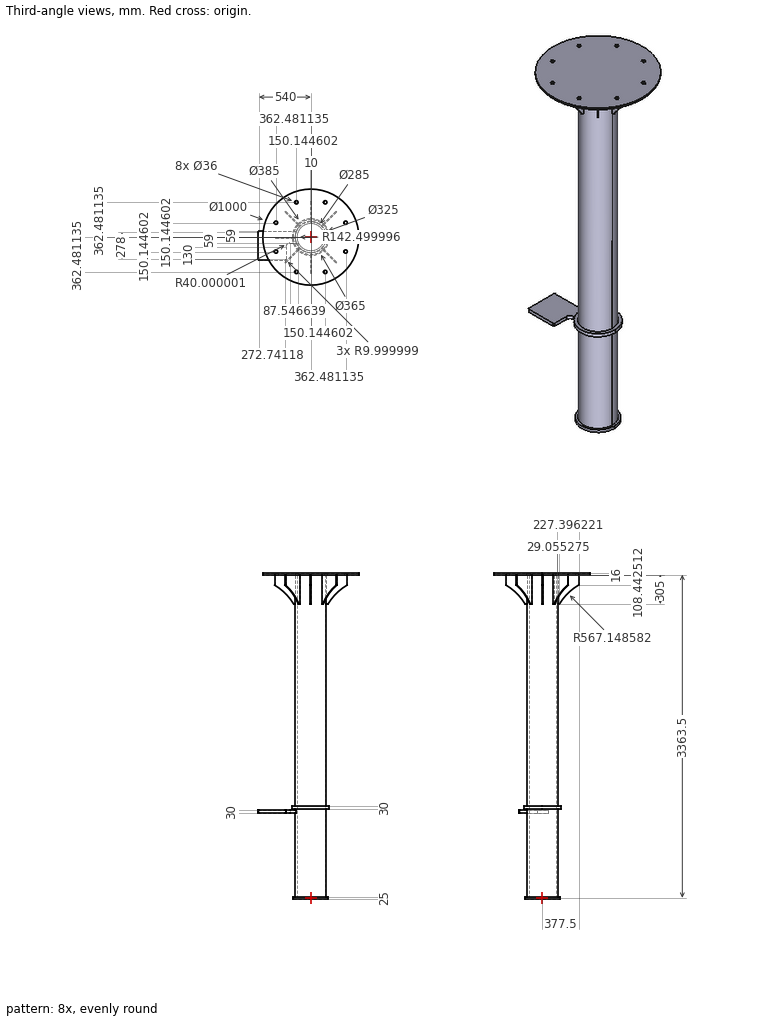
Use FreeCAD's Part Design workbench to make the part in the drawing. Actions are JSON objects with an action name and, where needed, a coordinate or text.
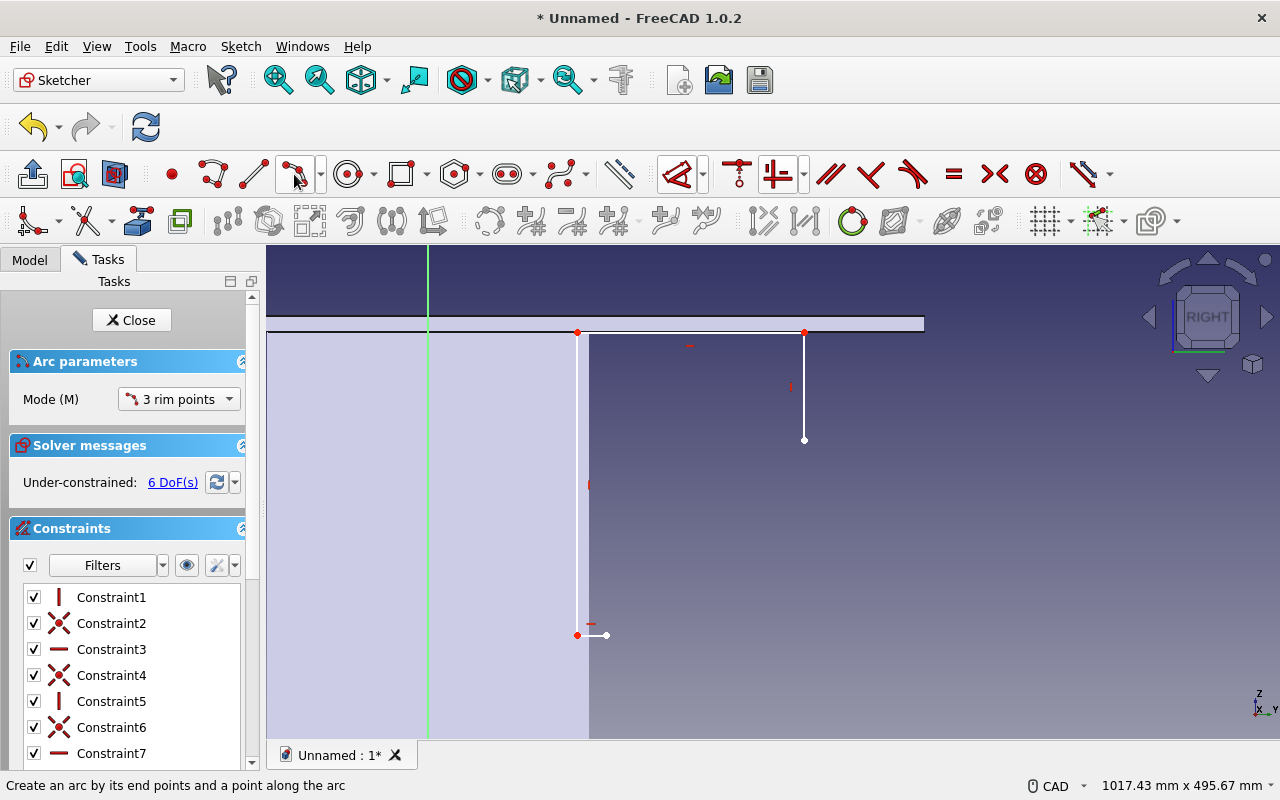
{"action": "left_click", "coordinate": [606, 636]}
{"action": "left_click", "coordinate": [804, 441]}
{"action": "left_click", "coordinate": [693, 525]}
{"action": "key", "text": "Escape"}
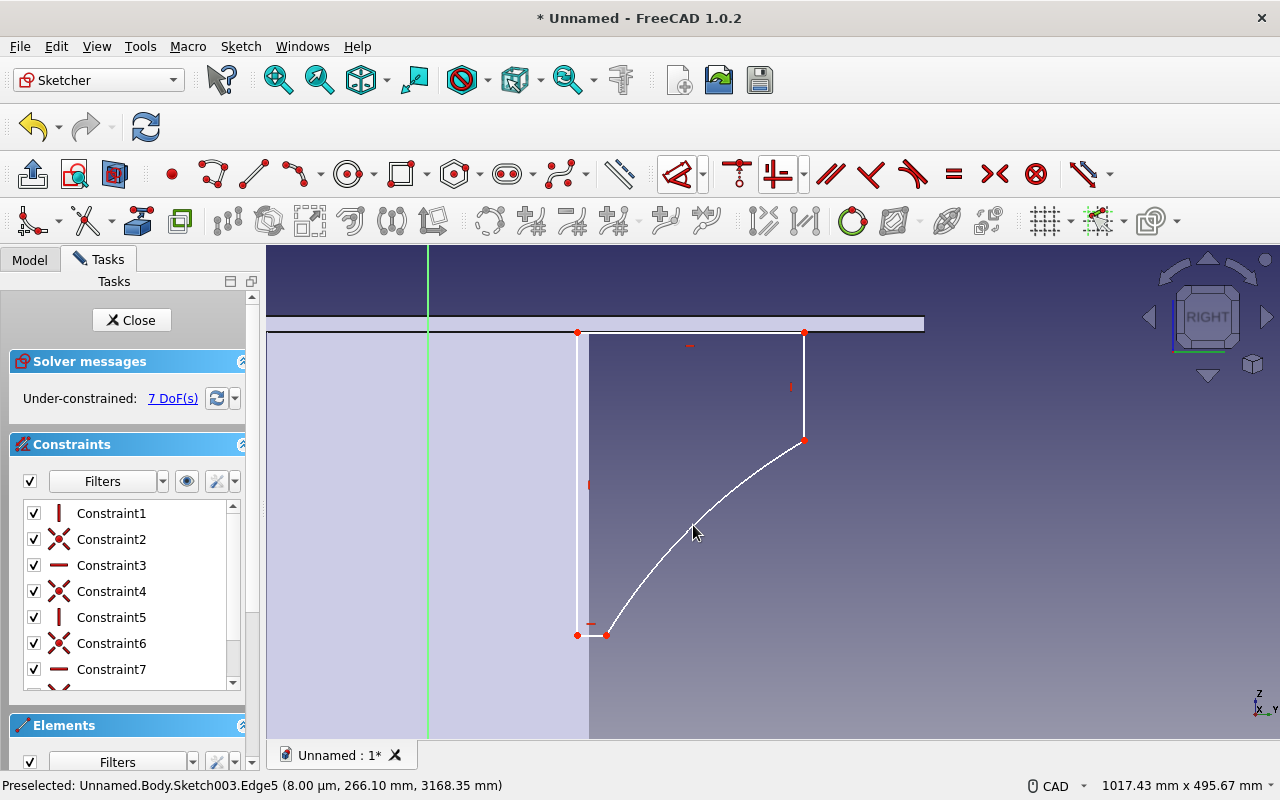
{"action": "left_click", "coordinate": [735, 489]}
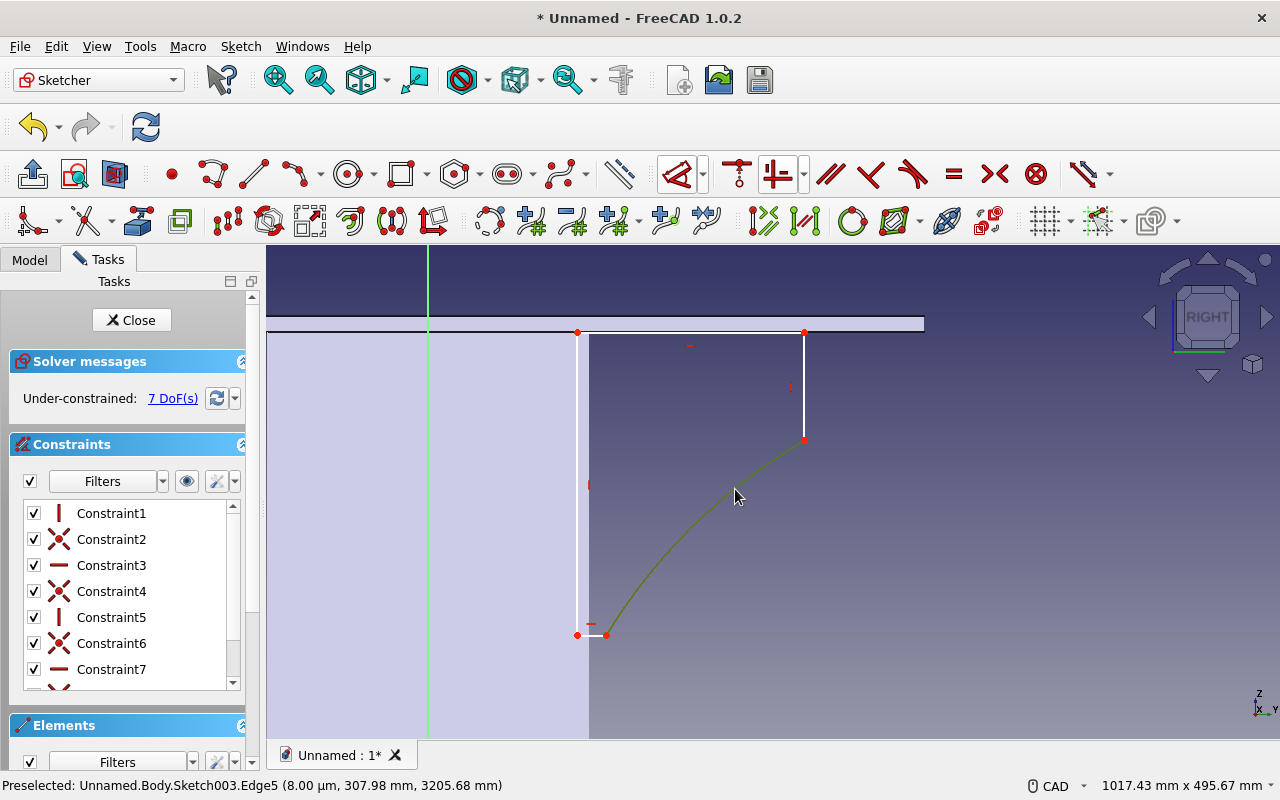
{"action": "left_click", "coordinate": [702, 174]}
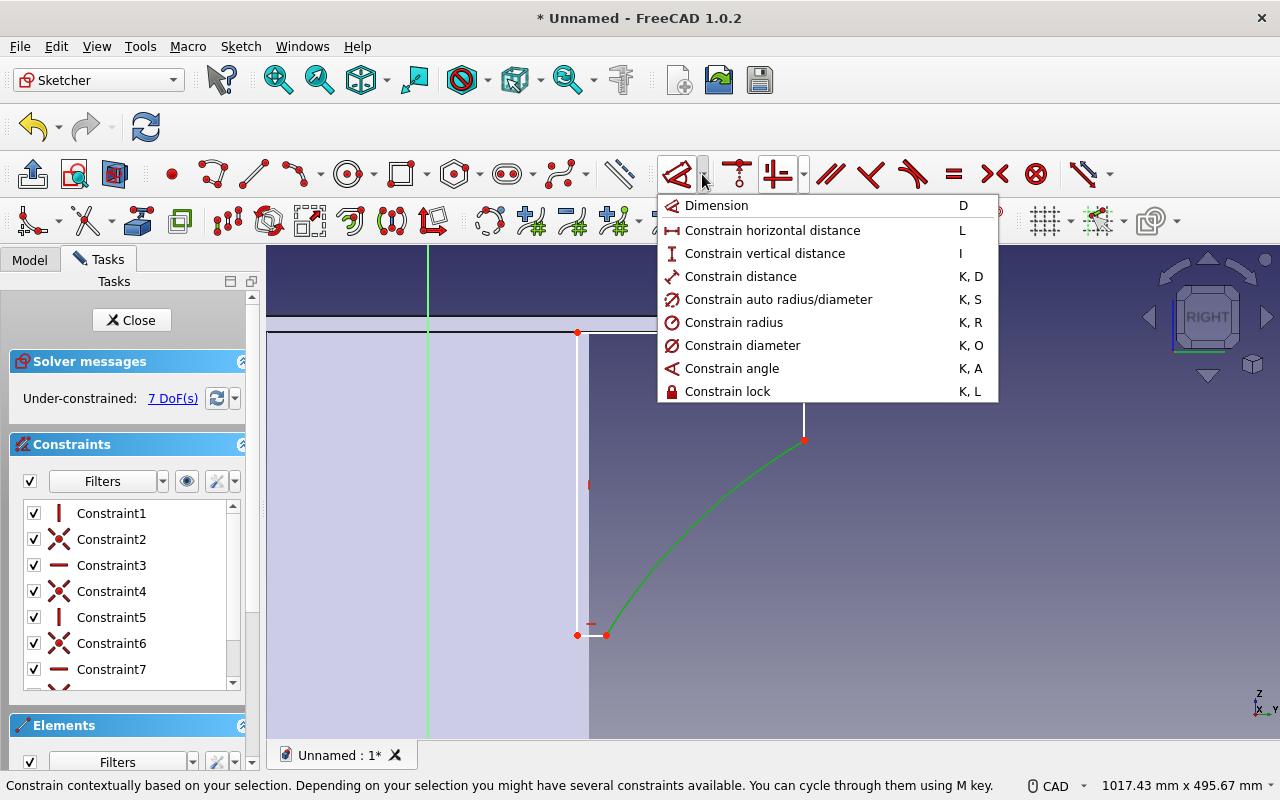
{"action": "left_click", "coordinate": [828, 322]}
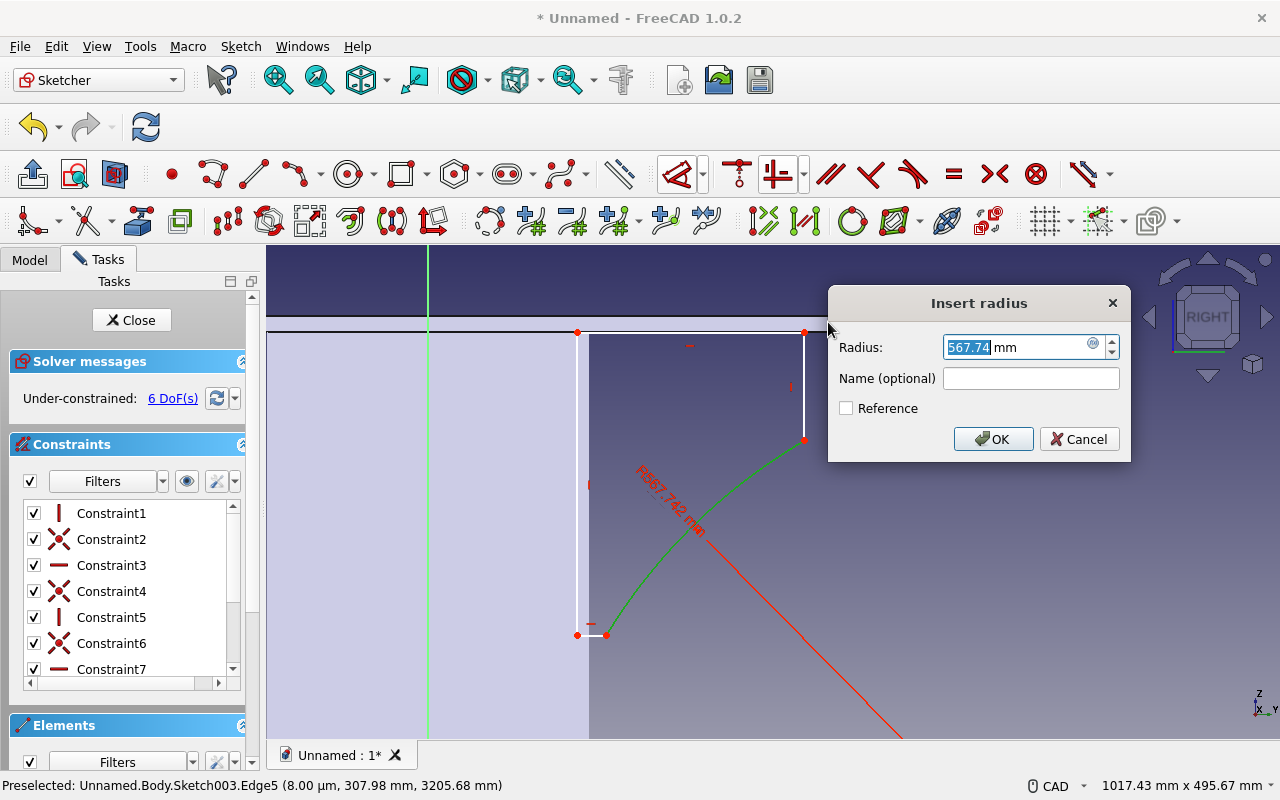
{"action": "type", "text": "567.148582"}
{"action": "key", "text": "Return"}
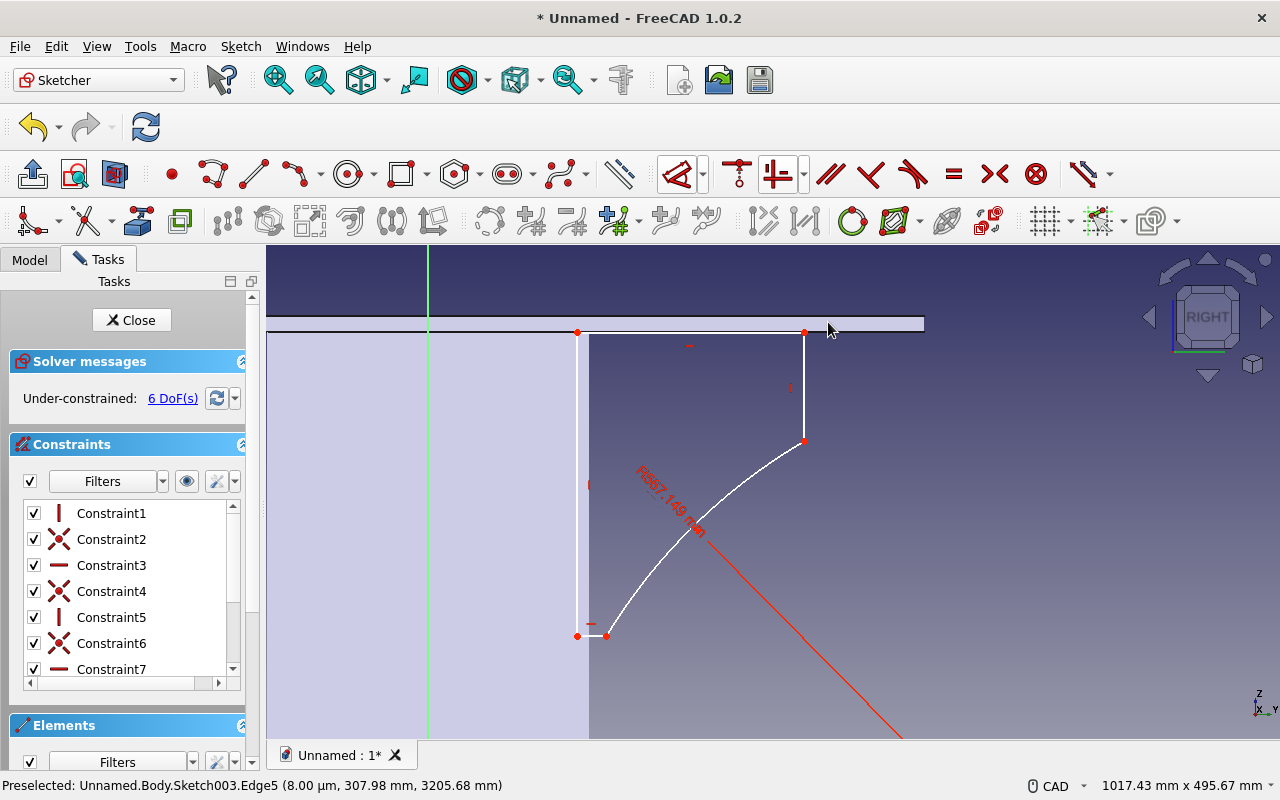
{"action": "left_click", "coordinate": [577, 424]}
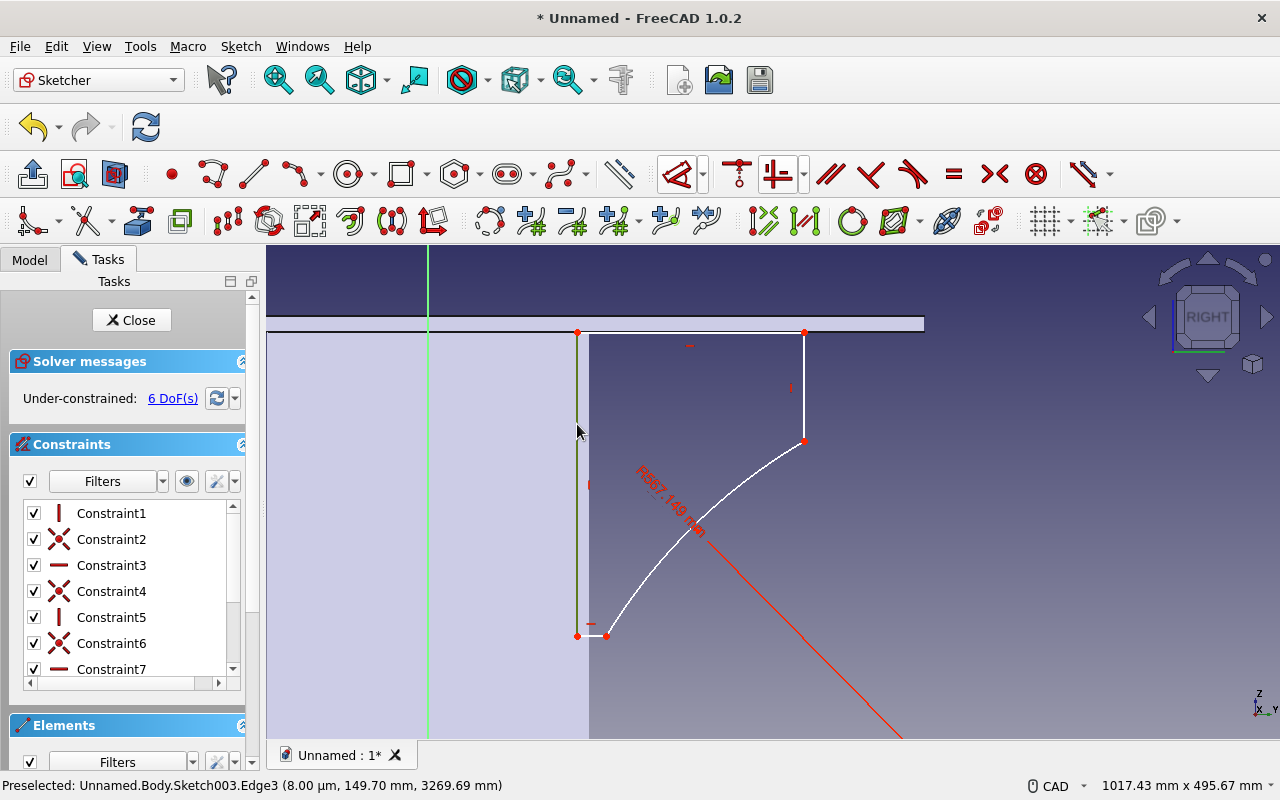
{"action": "key", "text": "i"}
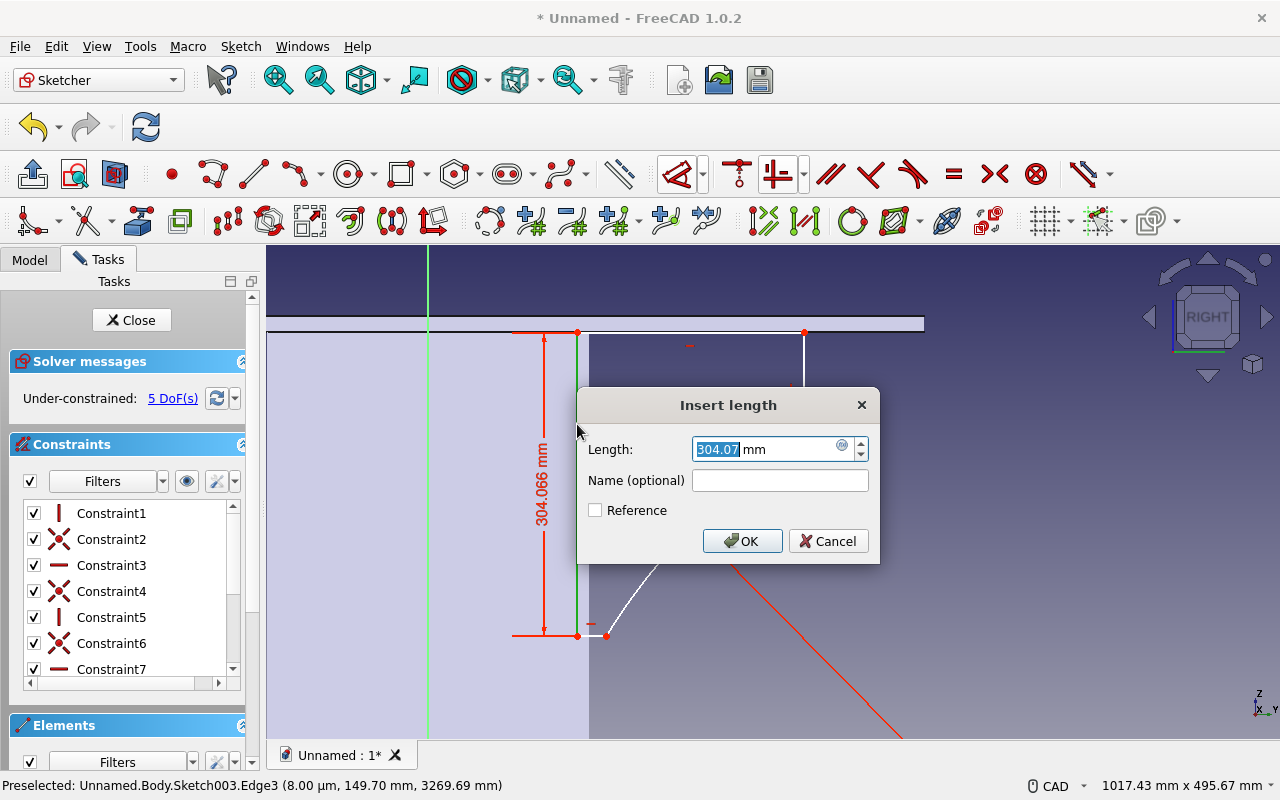
{"action": "type", "text": "305"}
{"action": "key", "text": "Return"}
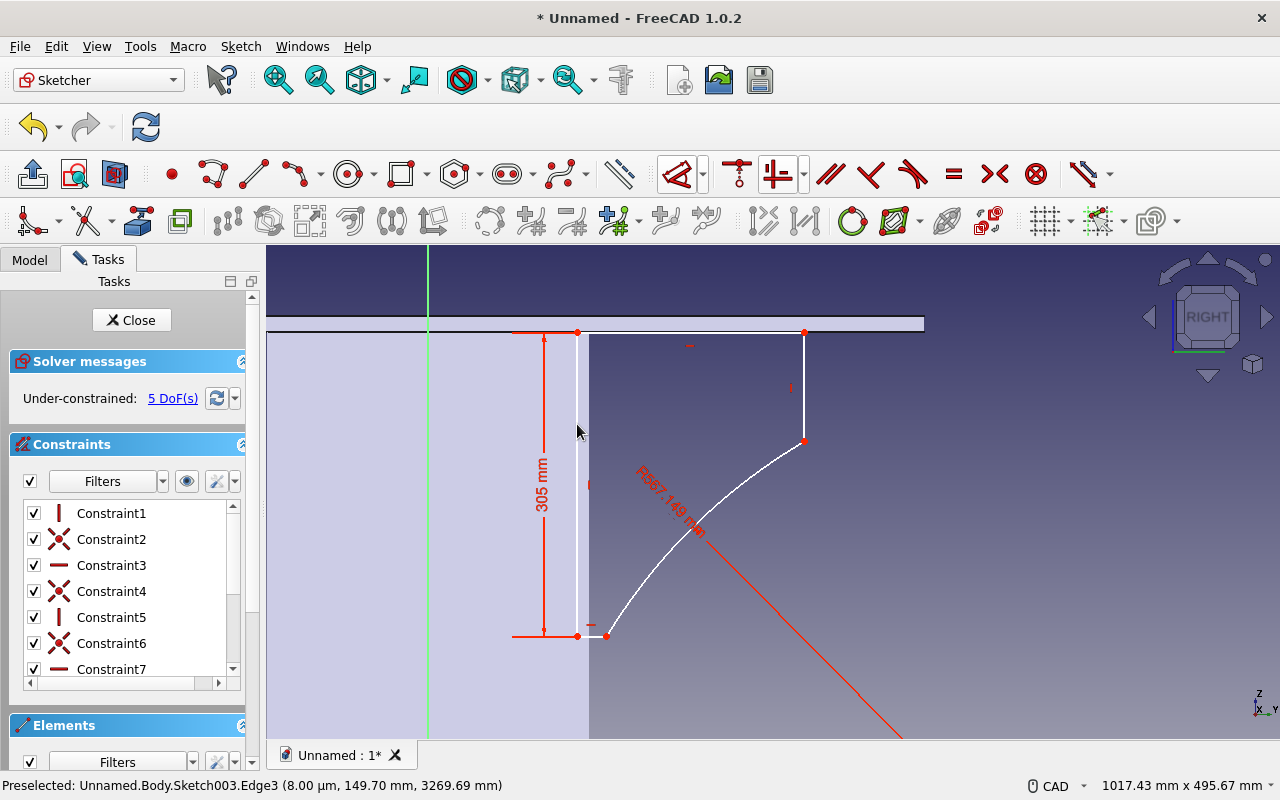
{"action": "left_click", "coordinate": [804, 442]}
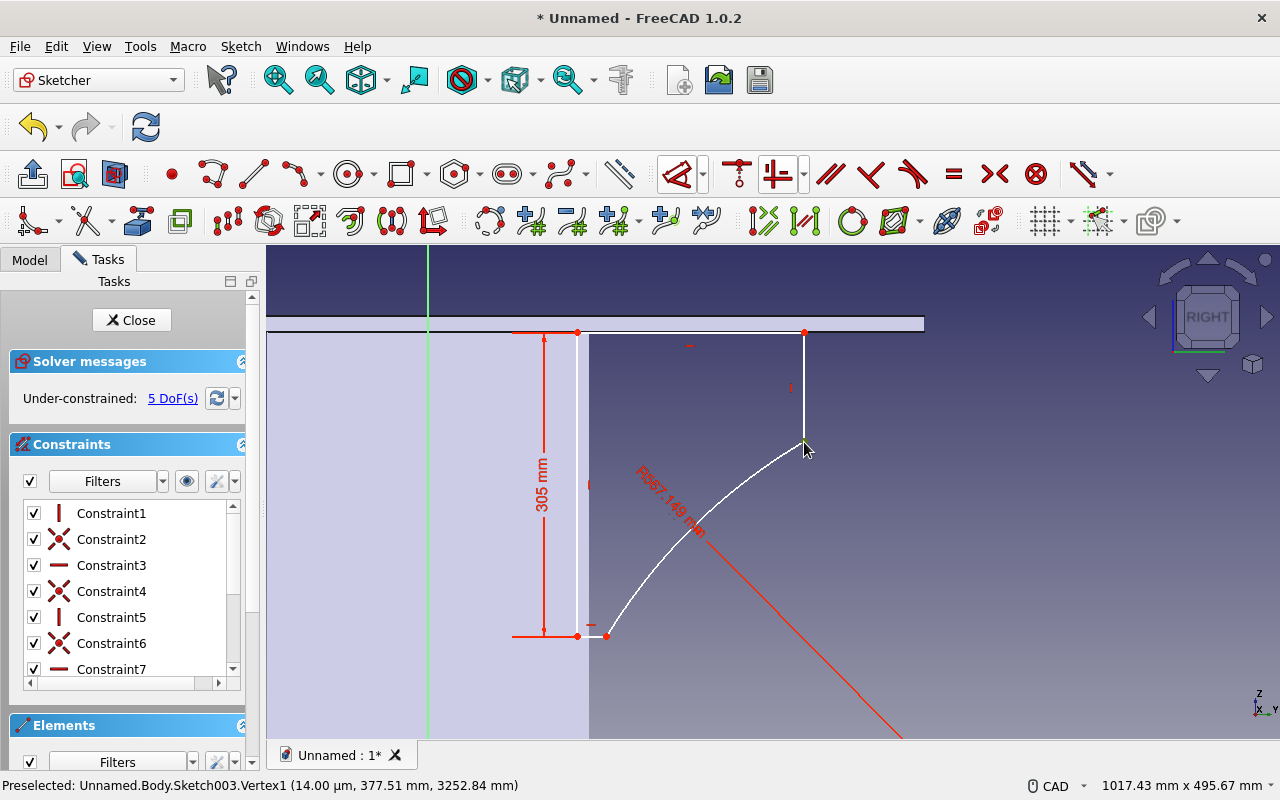
{"action": "left_click", "coordinate": [702, 174]}